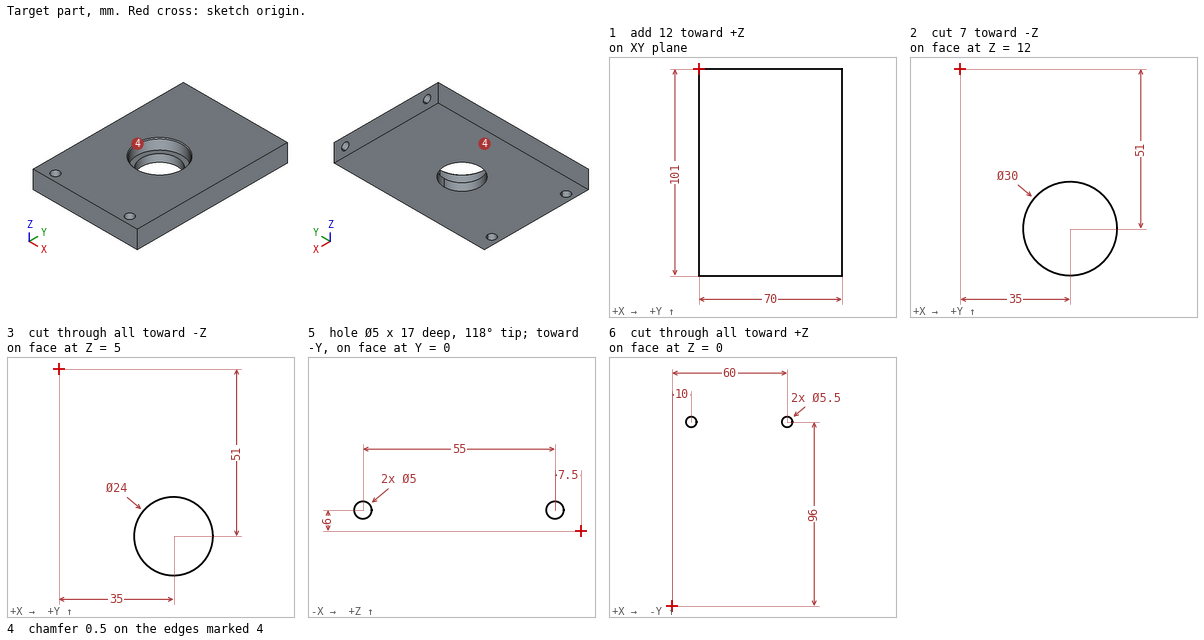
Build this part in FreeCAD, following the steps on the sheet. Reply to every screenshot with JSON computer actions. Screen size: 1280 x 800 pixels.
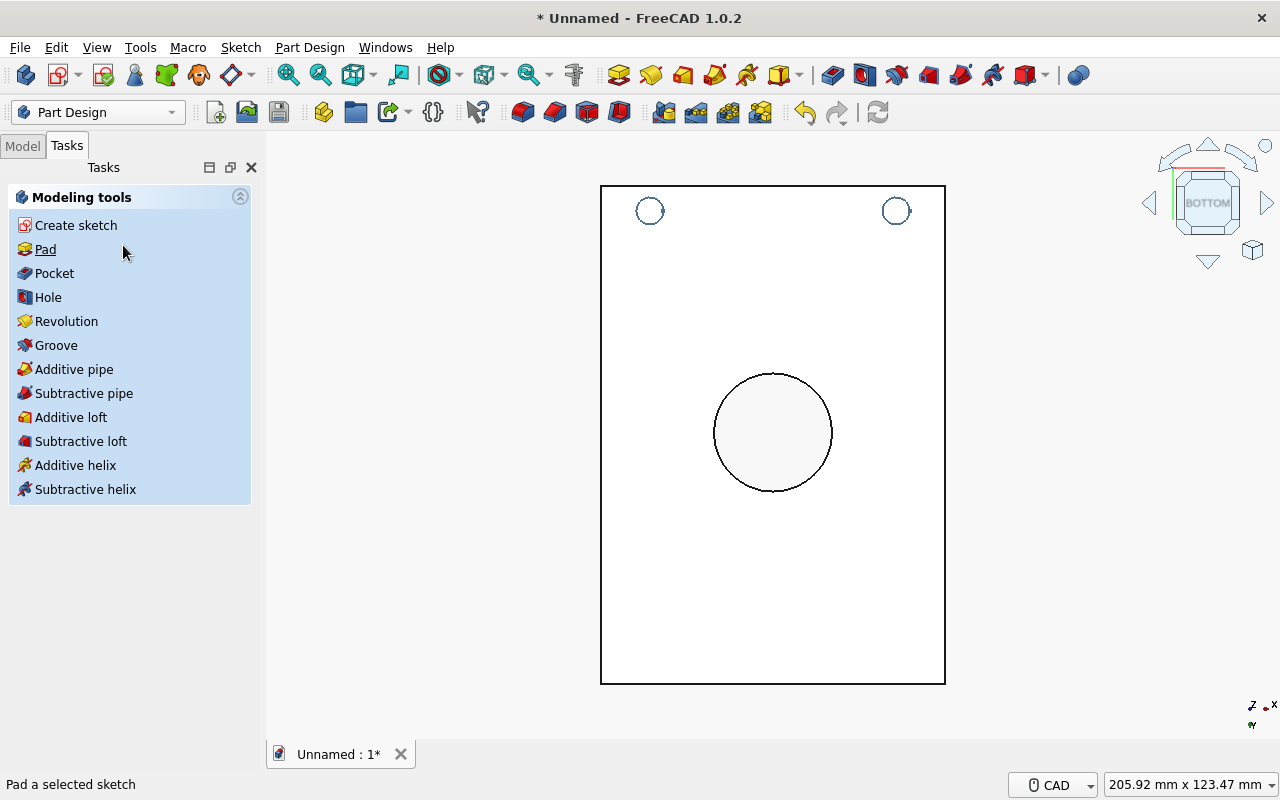
{"action": "left_click", "coordinate": [834, 76]}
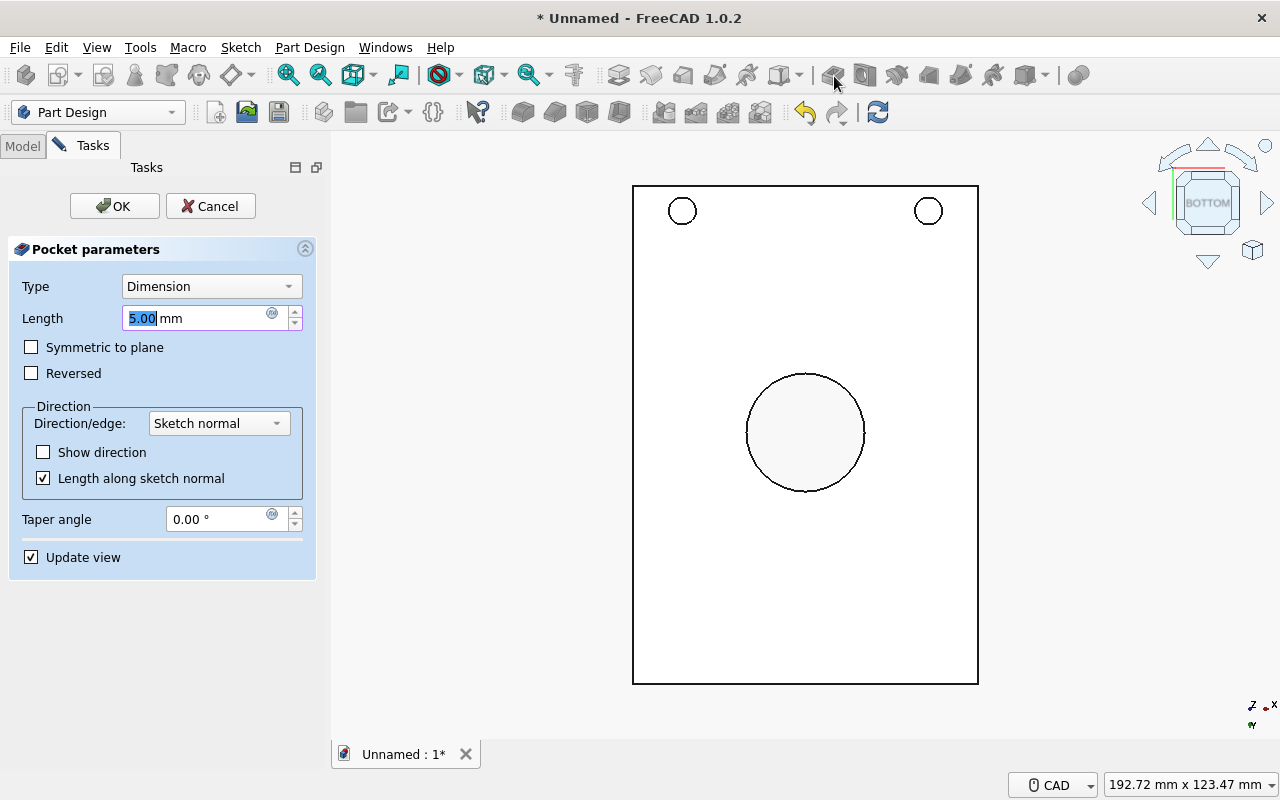
{"action": "left_click", "coordinate": [212, 286]}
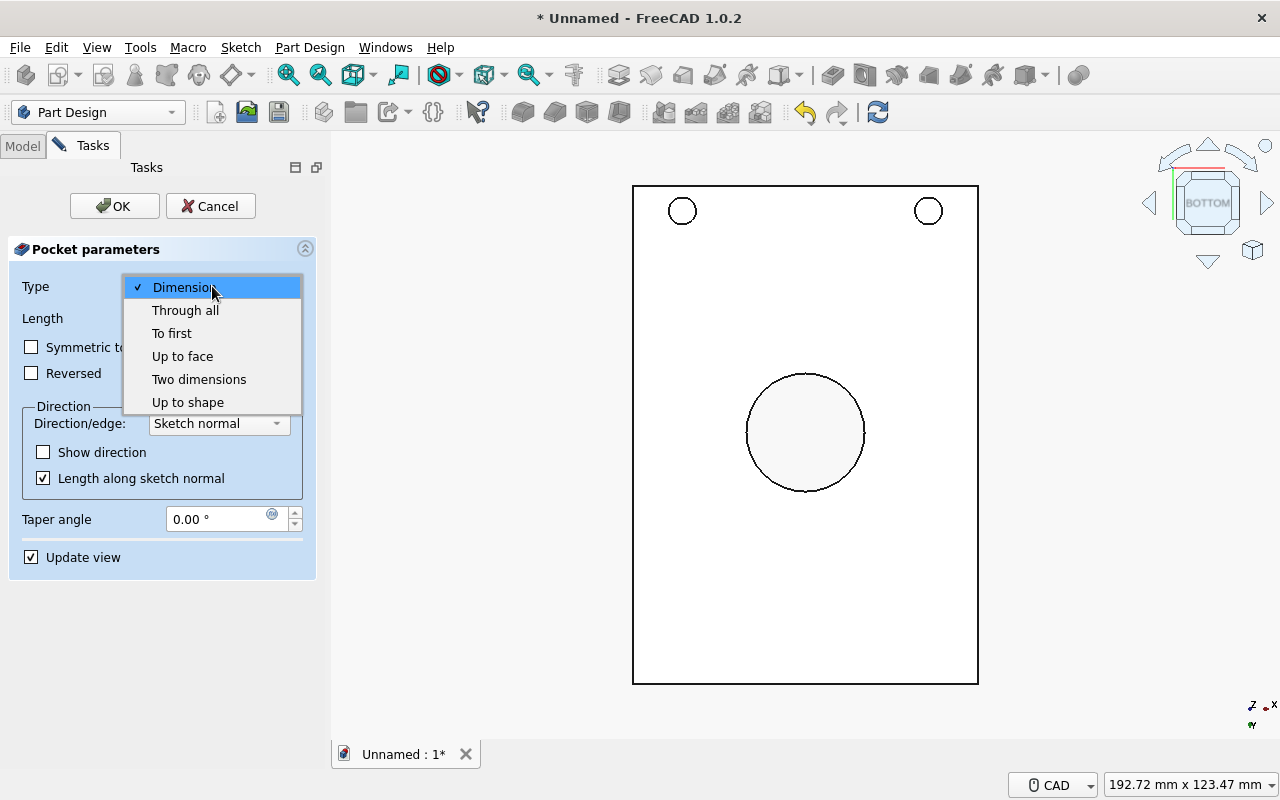
{"action": "left_click", "coordinate": [212, 310]}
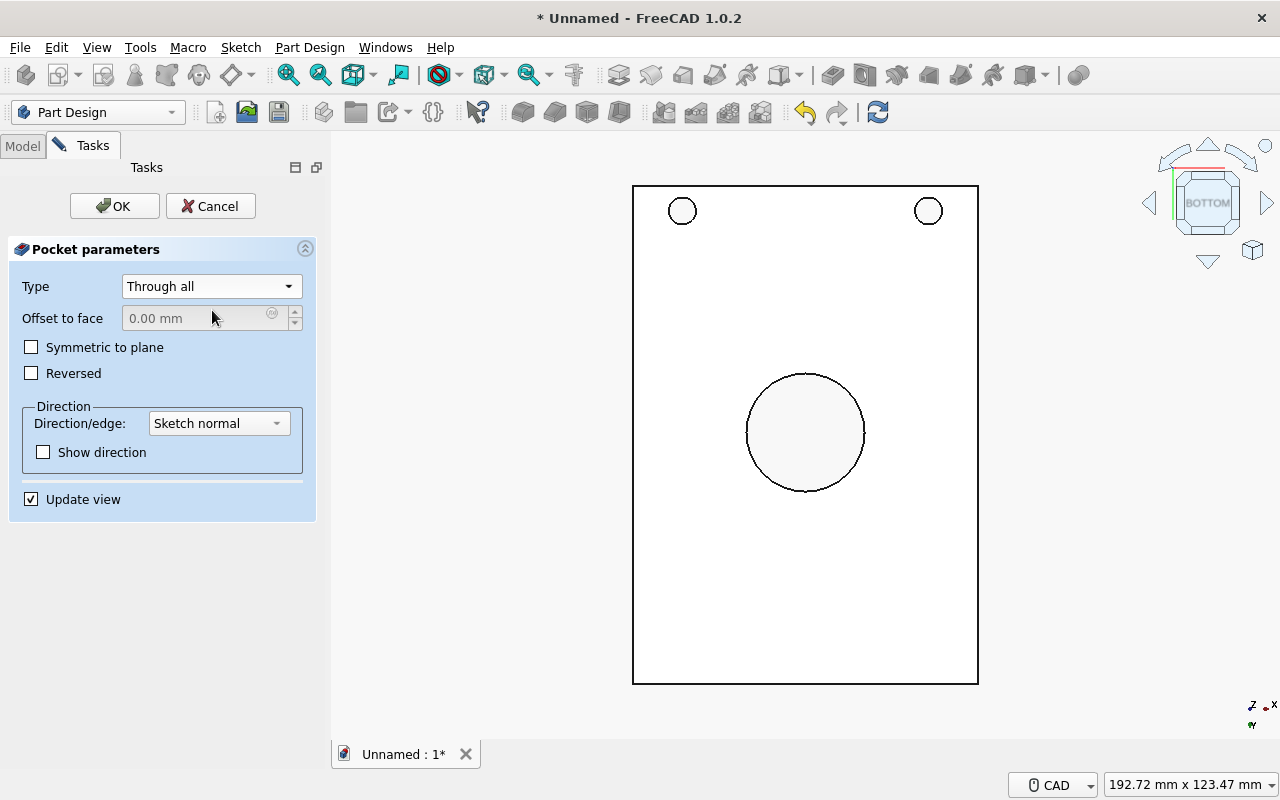
{"action": "left_click", "coordinate": [115, 206]}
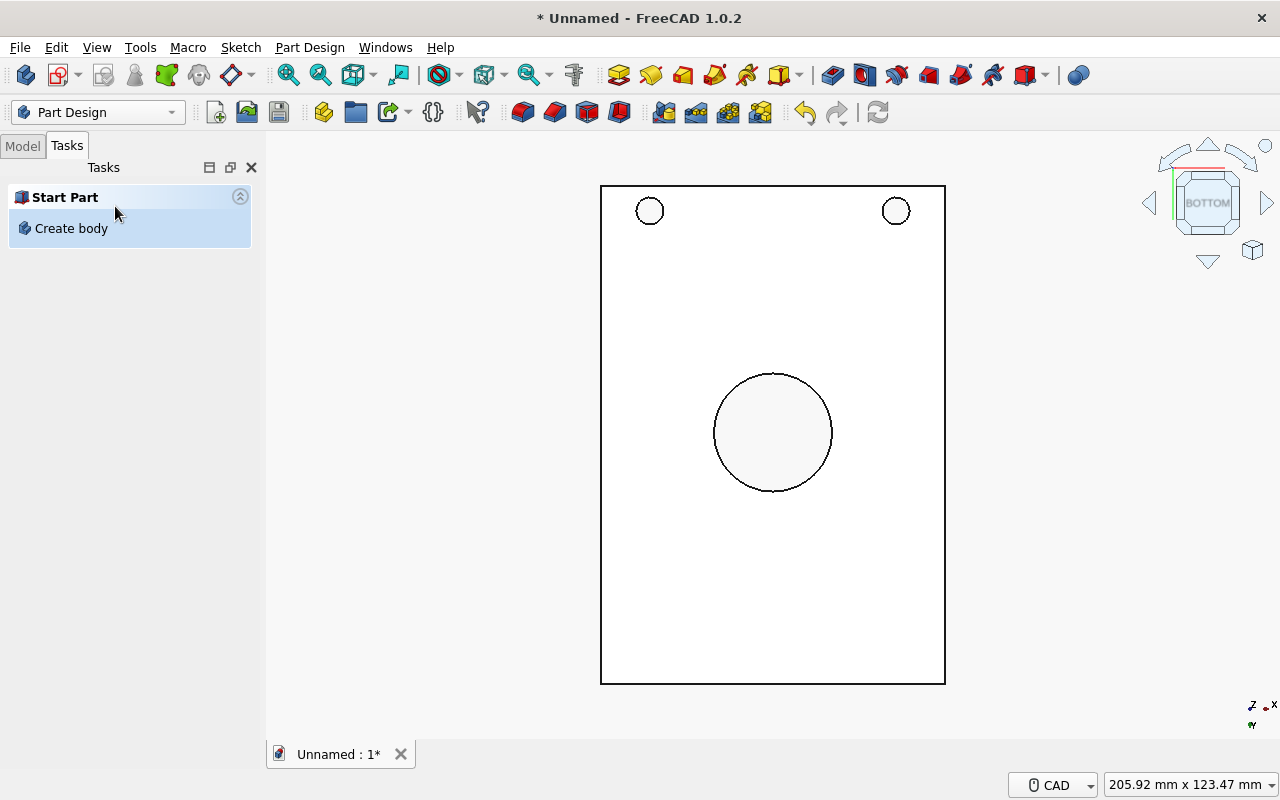
{"action": "key", "text": "0"}